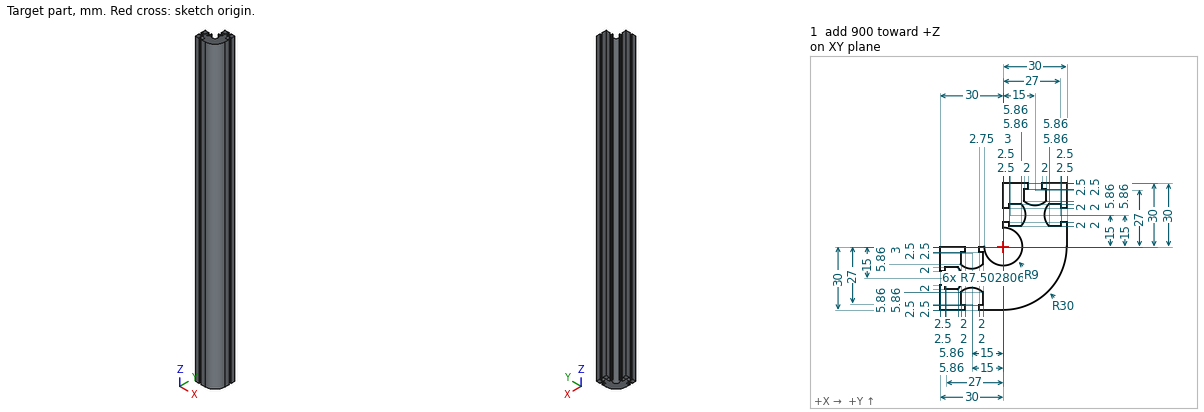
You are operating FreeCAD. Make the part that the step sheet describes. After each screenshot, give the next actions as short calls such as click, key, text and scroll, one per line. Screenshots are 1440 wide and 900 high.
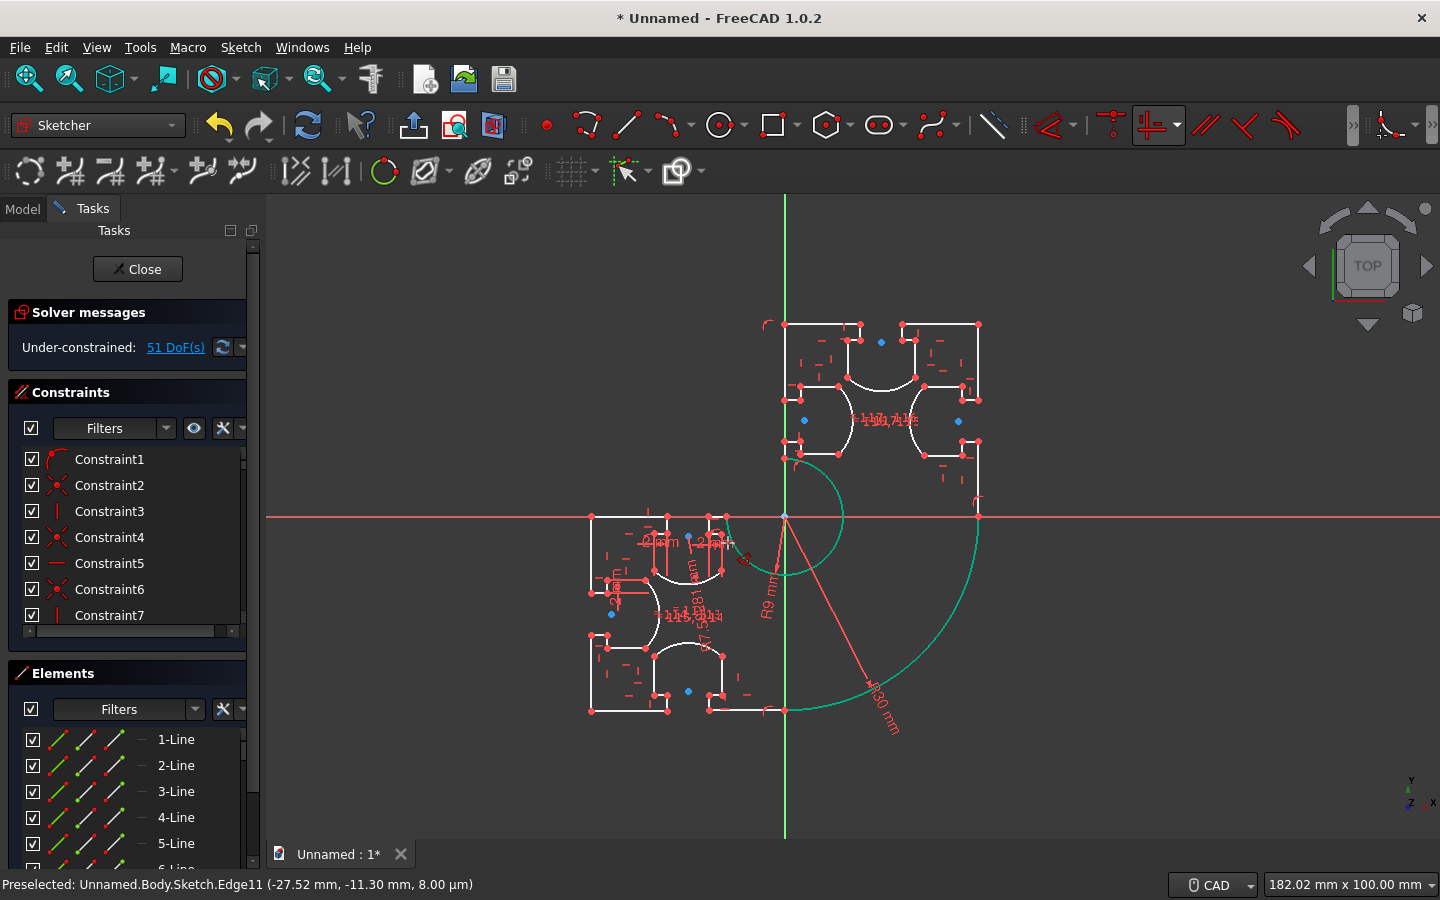
scroll(607, 644, up, 7)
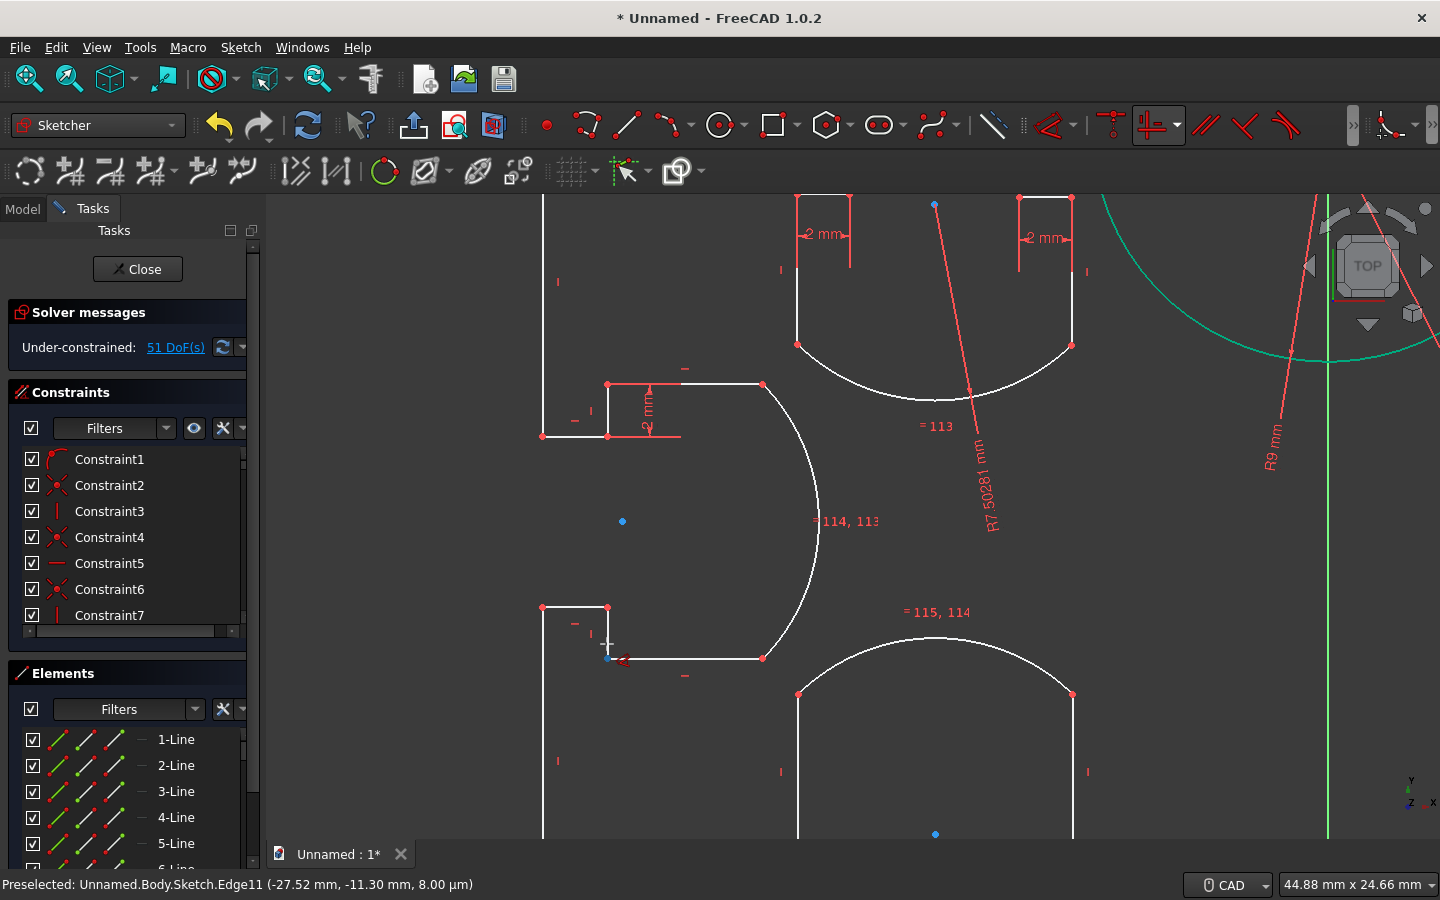
click(608, 643)
click(574, 633)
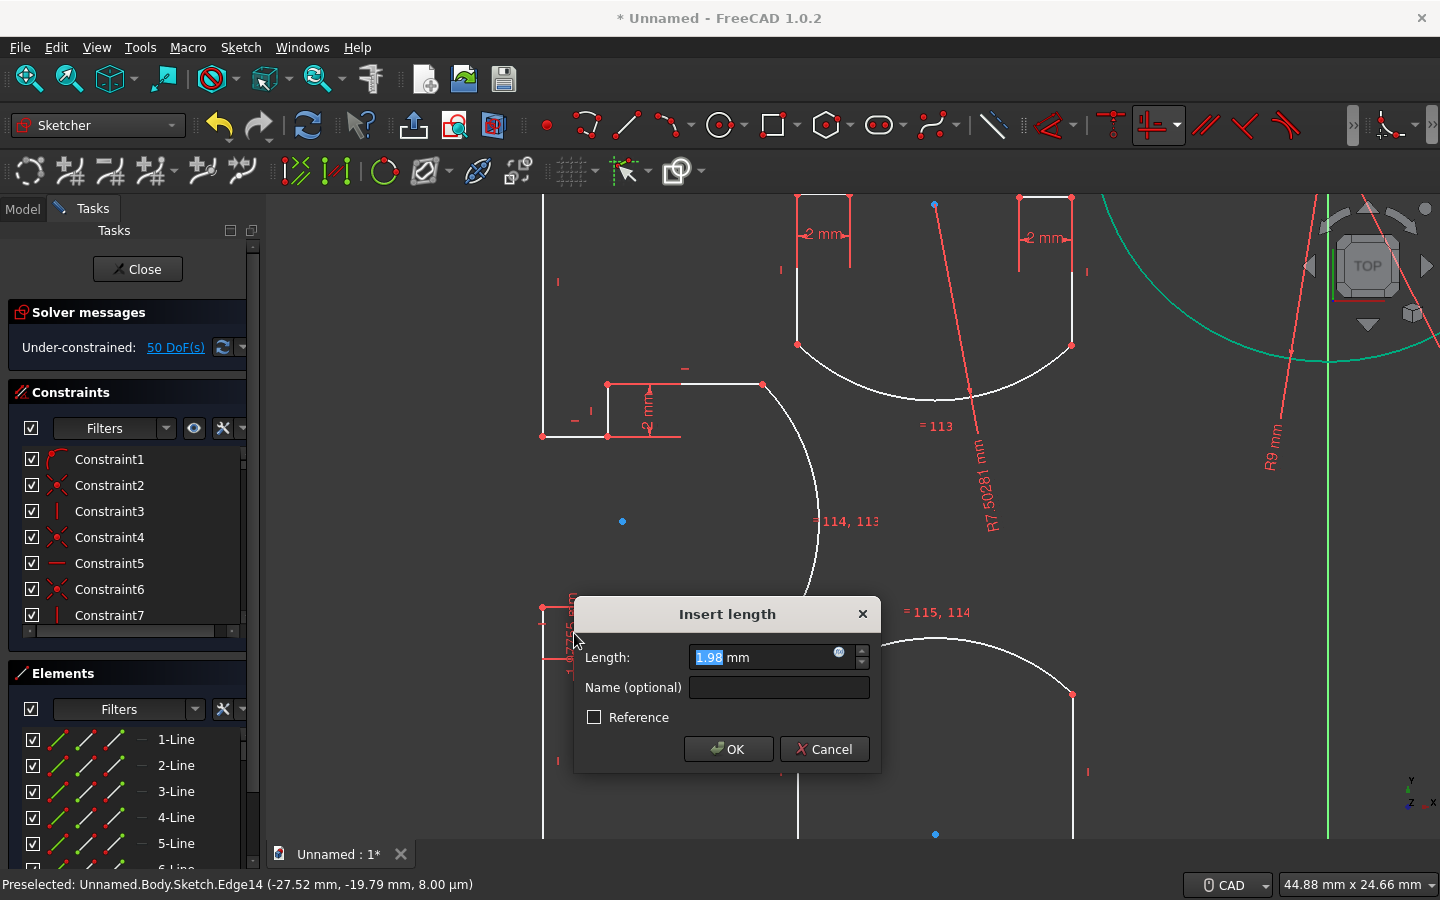
text(2)
key(Return)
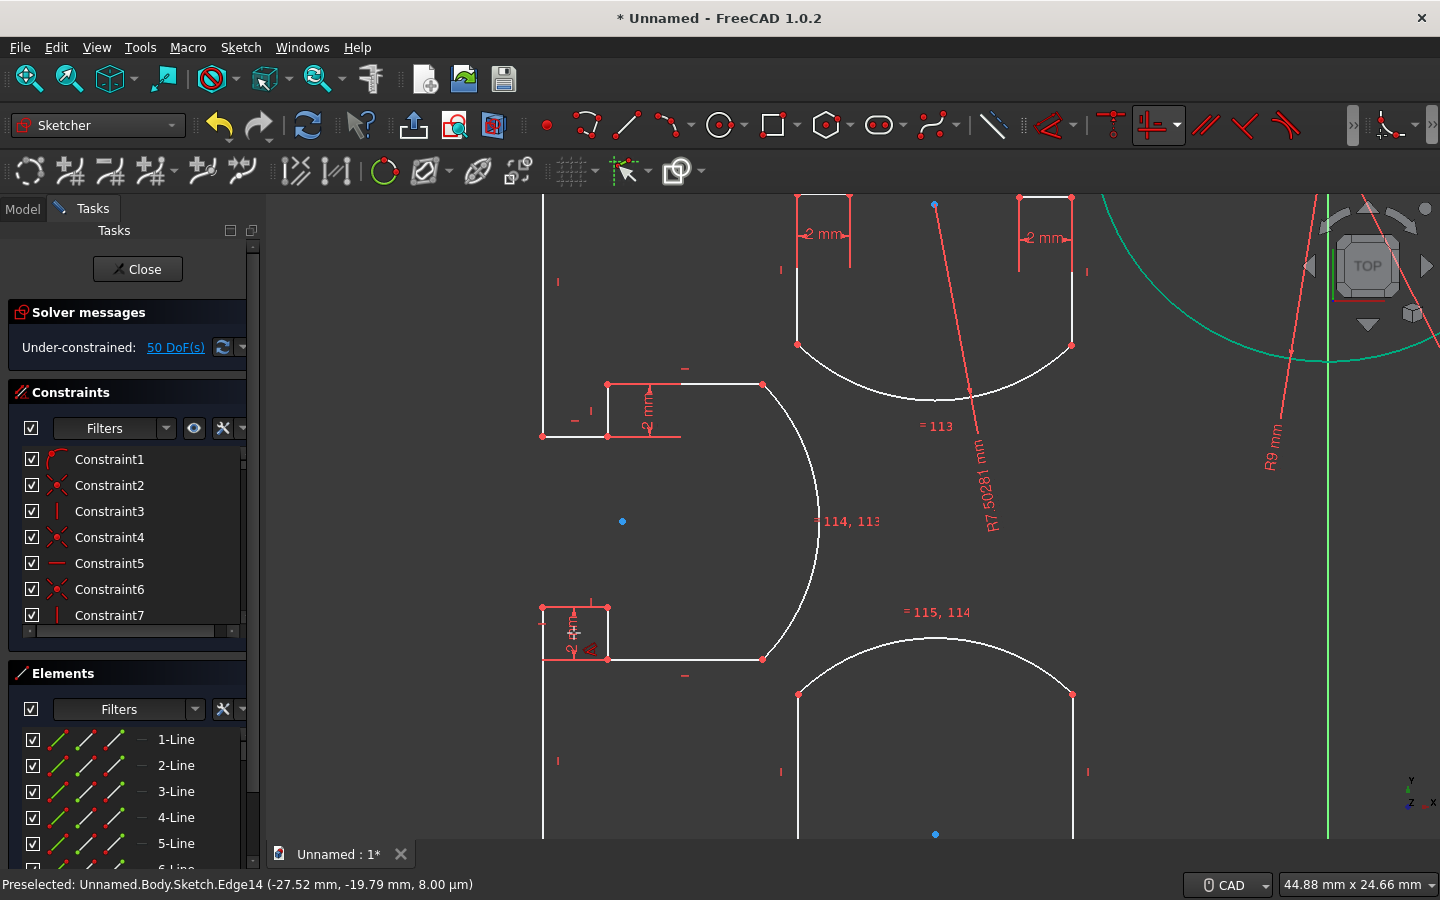
scroll(607, 644, down, 7)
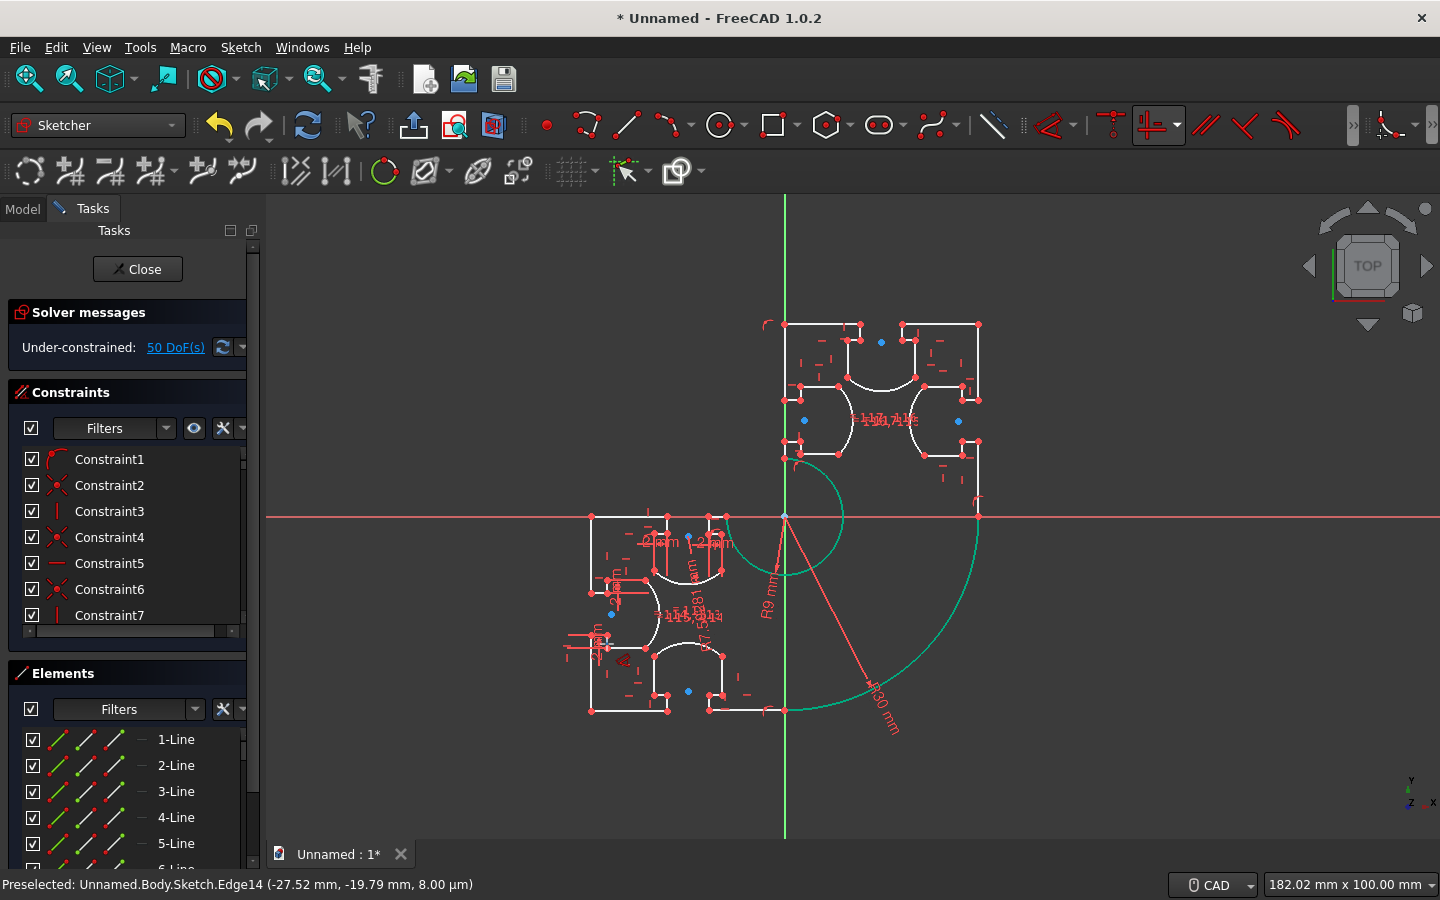
scroll(663, 695, up, 7)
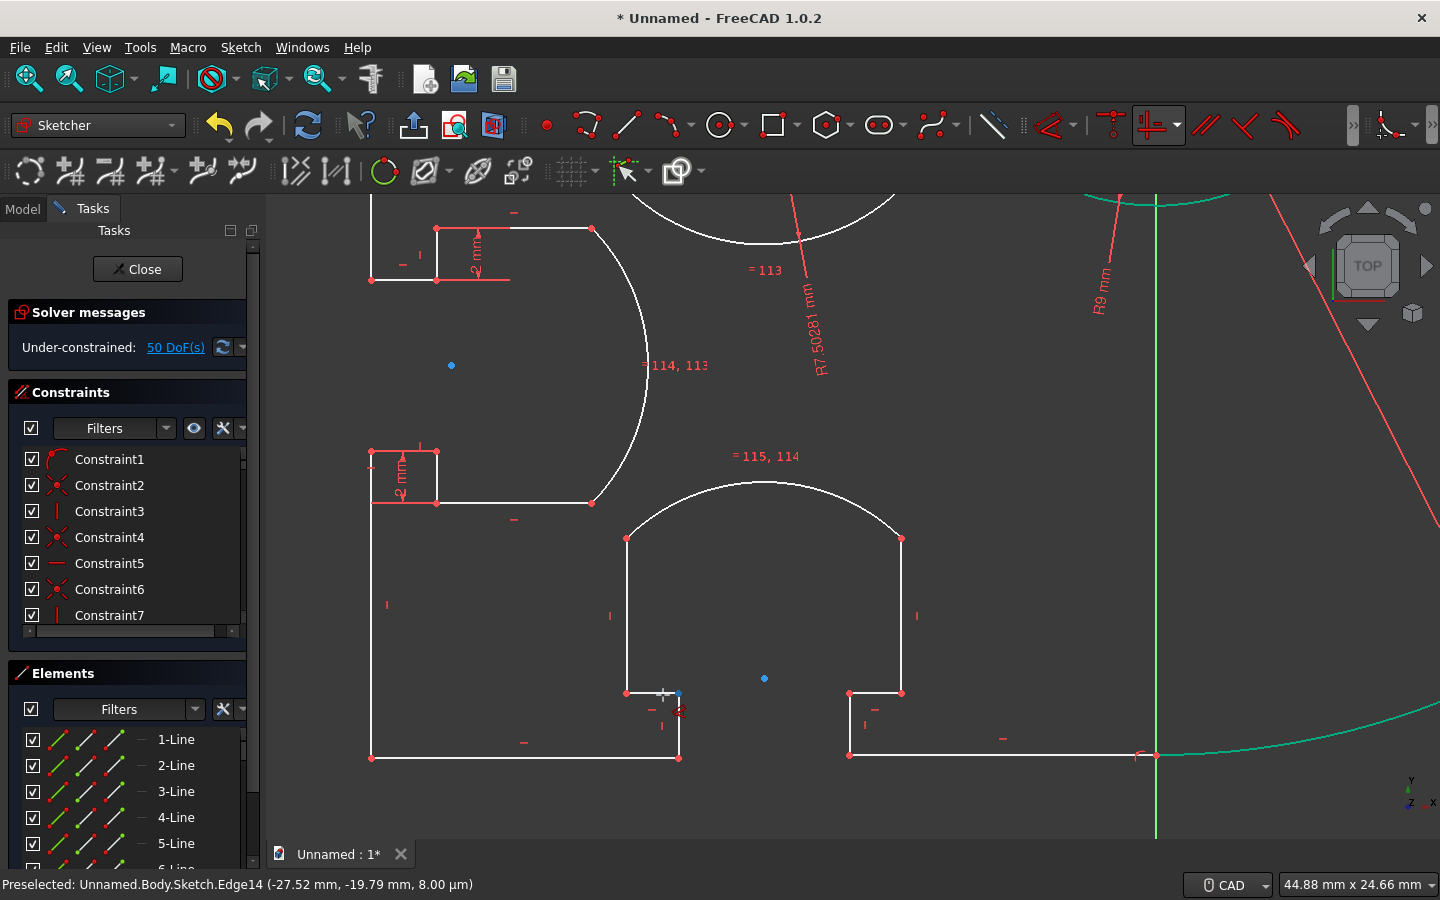
click(663, 693)
click(653, 727)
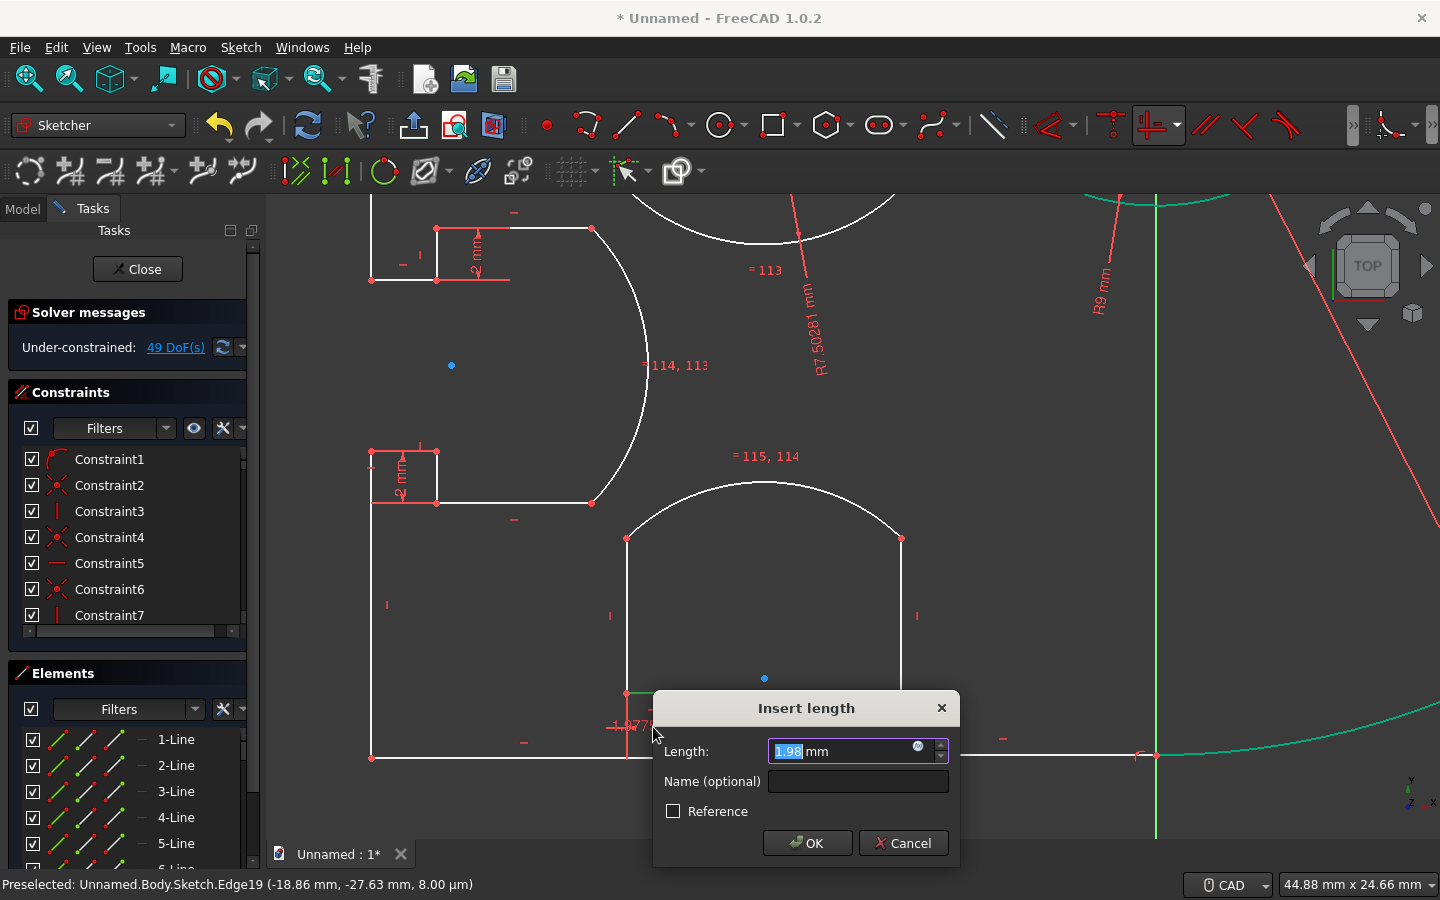
text(2)
key(Return)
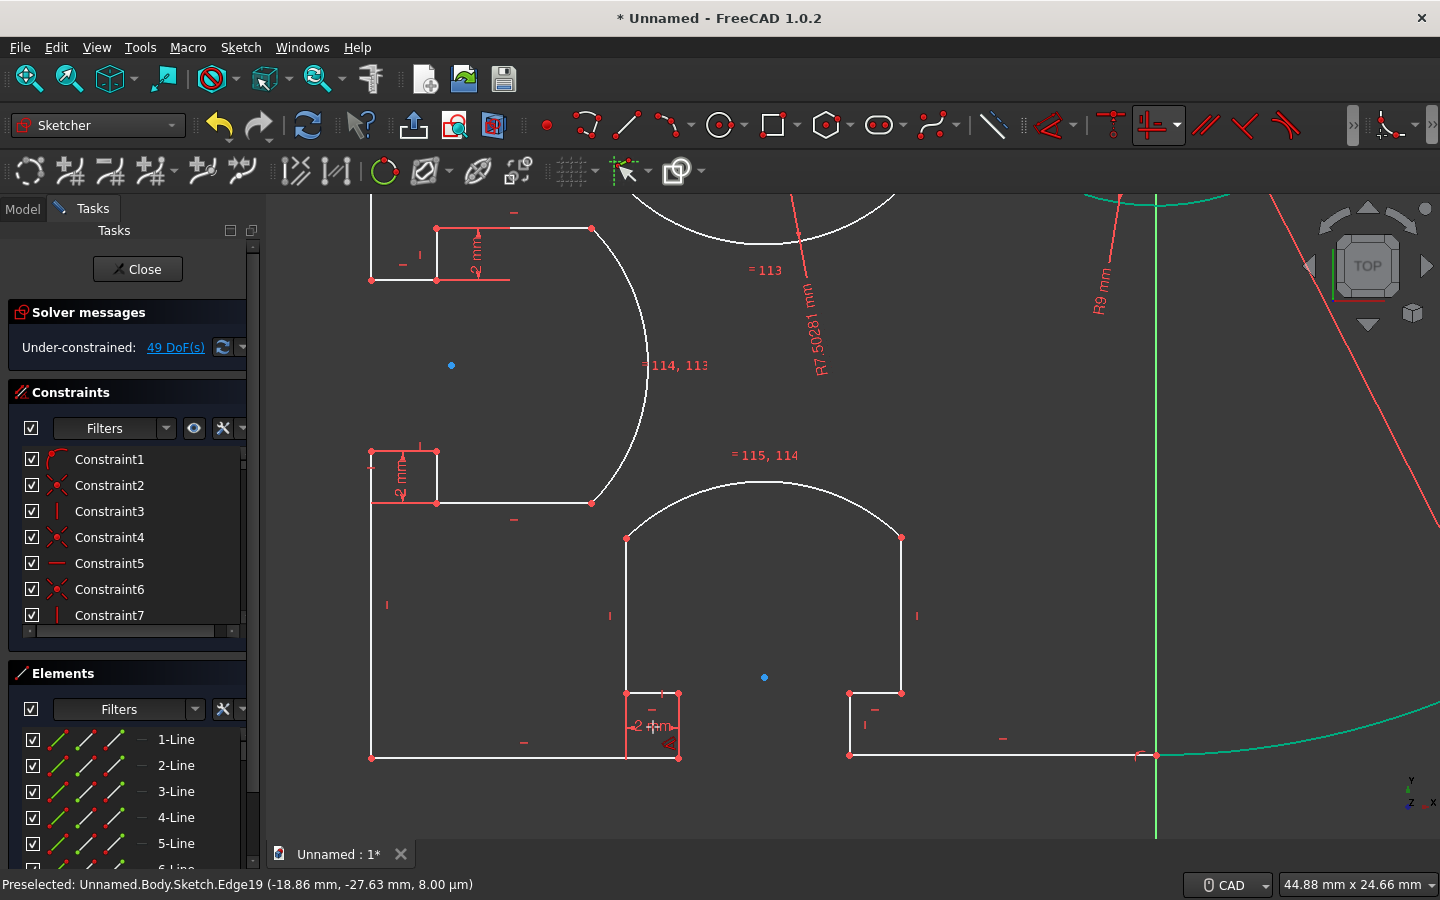
click(886, 693)
click(876, 727)